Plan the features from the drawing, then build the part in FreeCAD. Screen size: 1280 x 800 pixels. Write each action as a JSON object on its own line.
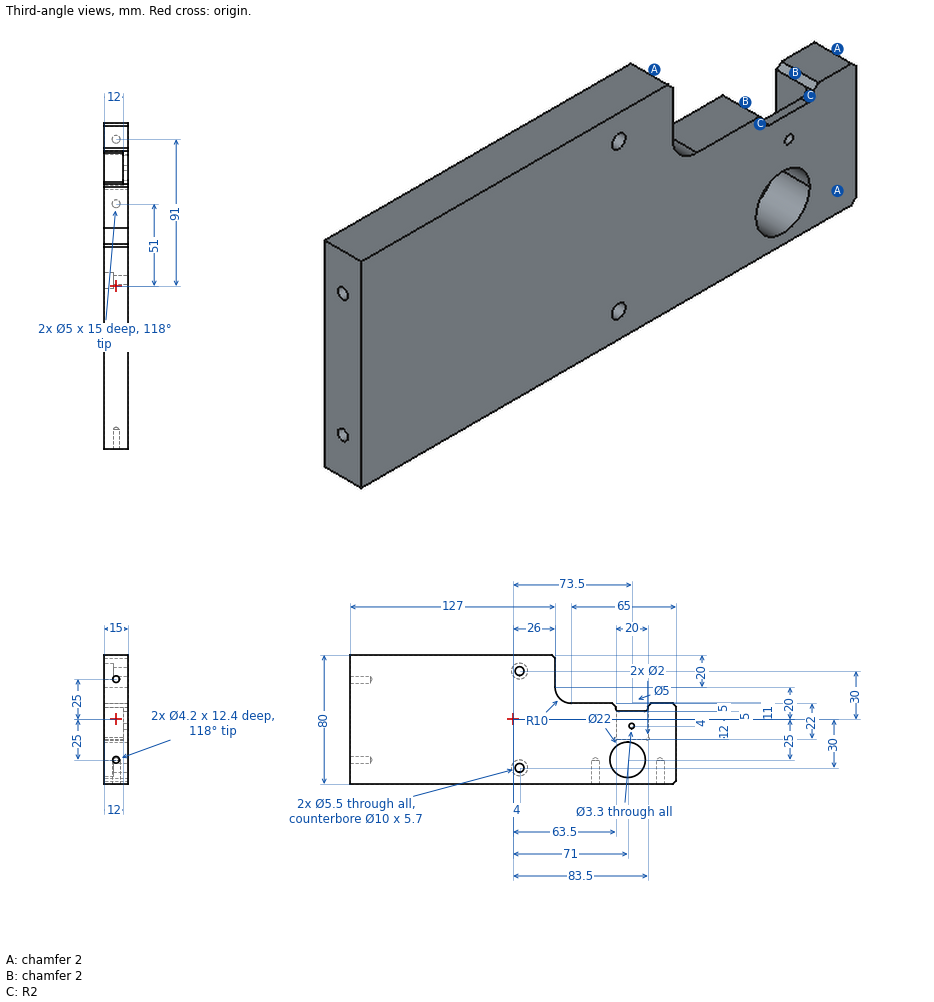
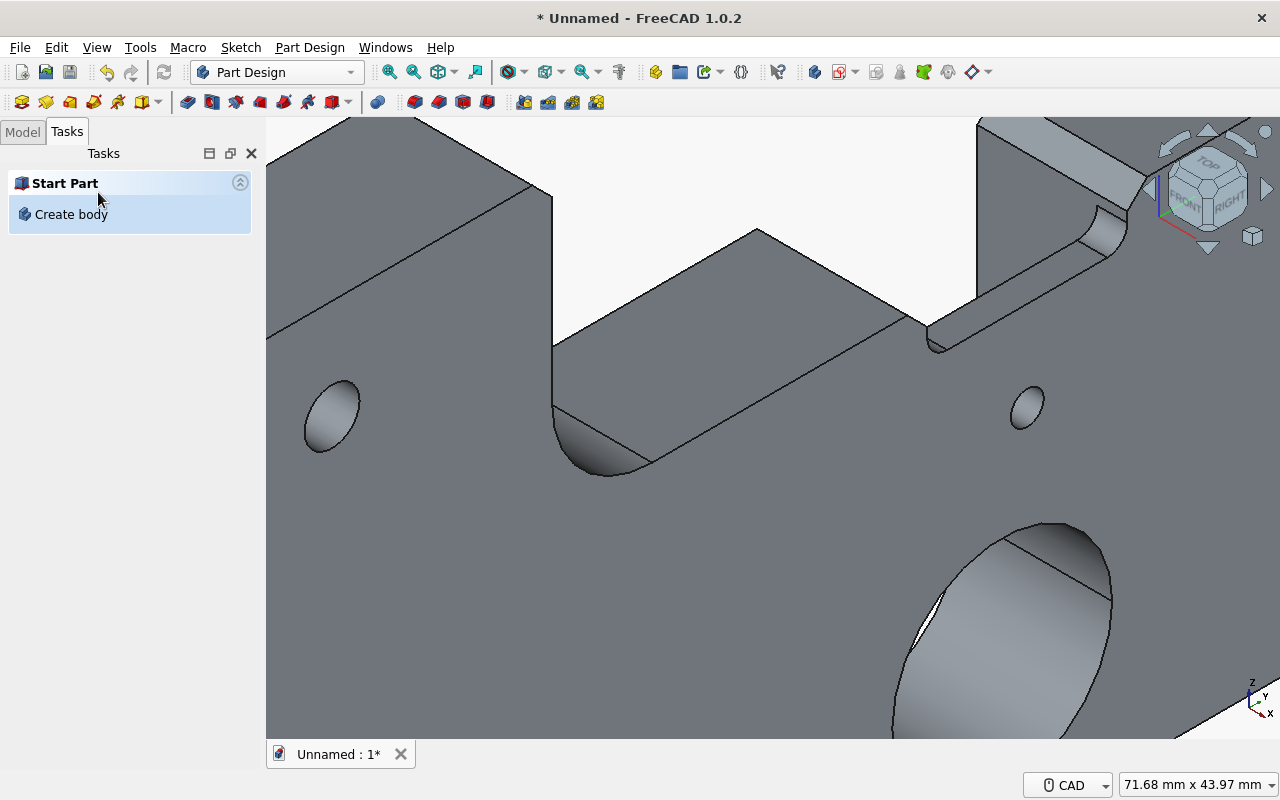
{"action": "left_click", "coordinate": [390, 72]}